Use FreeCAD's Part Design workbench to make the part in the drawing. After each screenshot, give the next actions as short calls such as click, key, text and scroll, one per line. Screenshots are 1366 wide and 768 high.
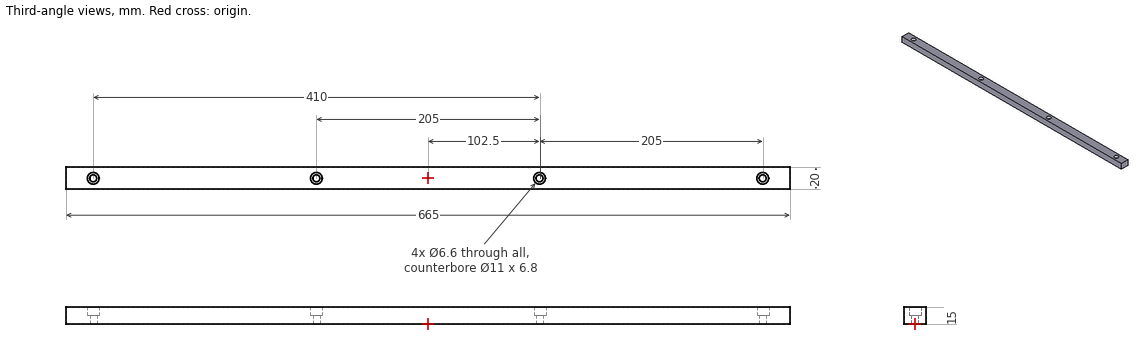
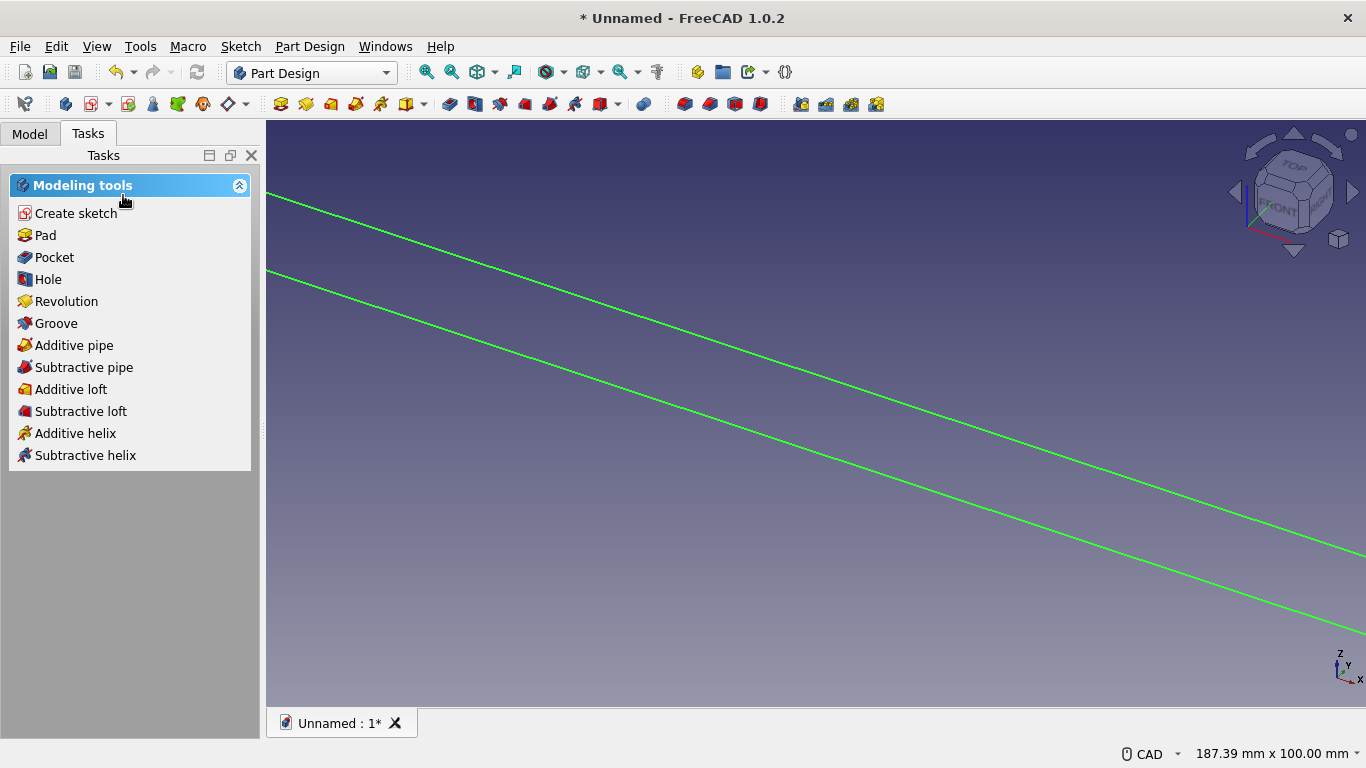
click(281, 104)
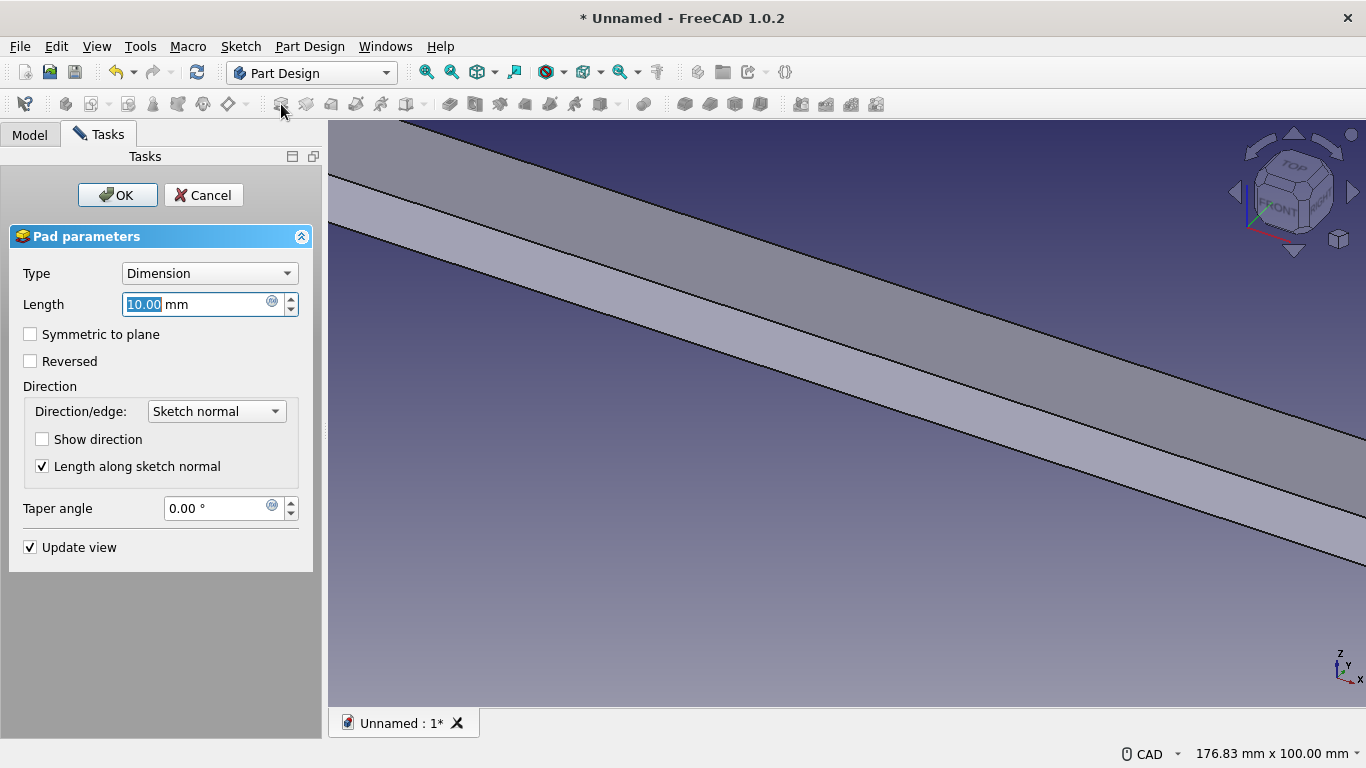
text(15)
key(Tab)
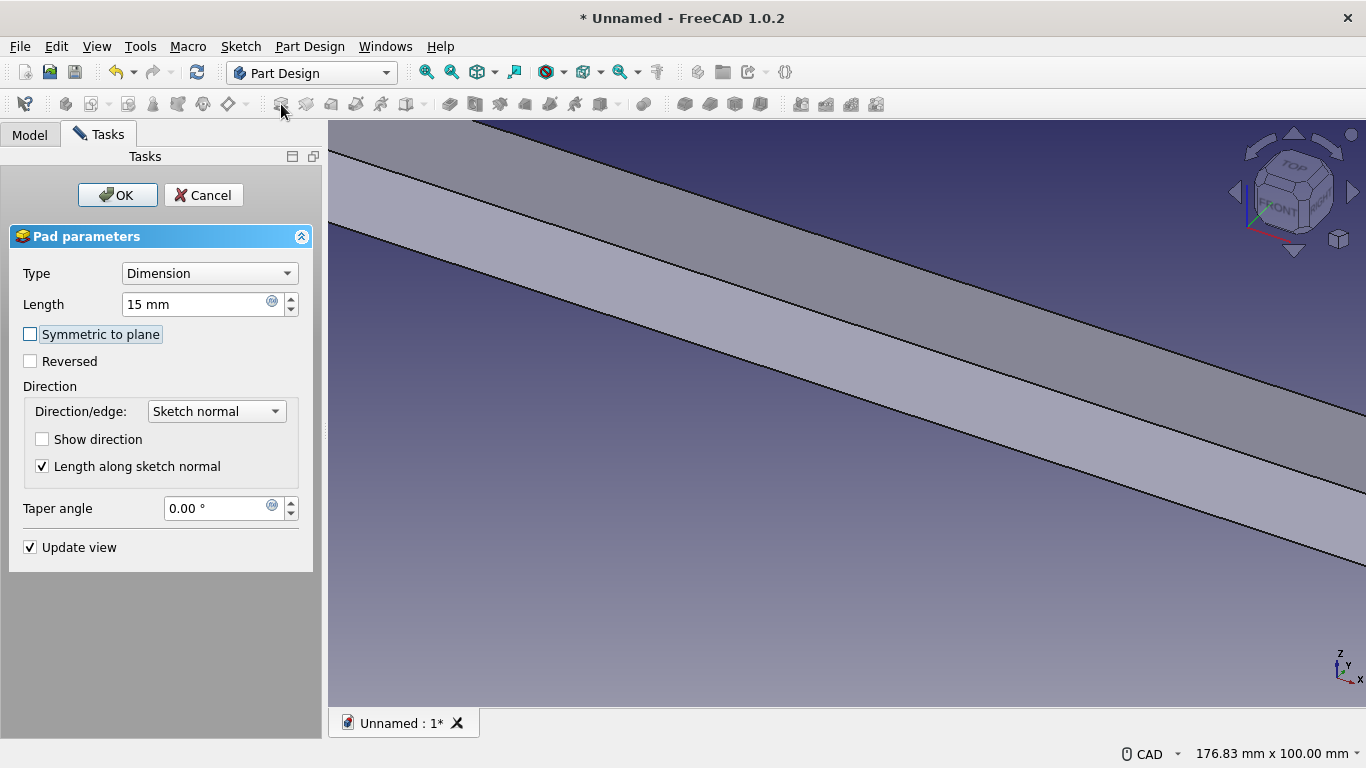
click(118, 195)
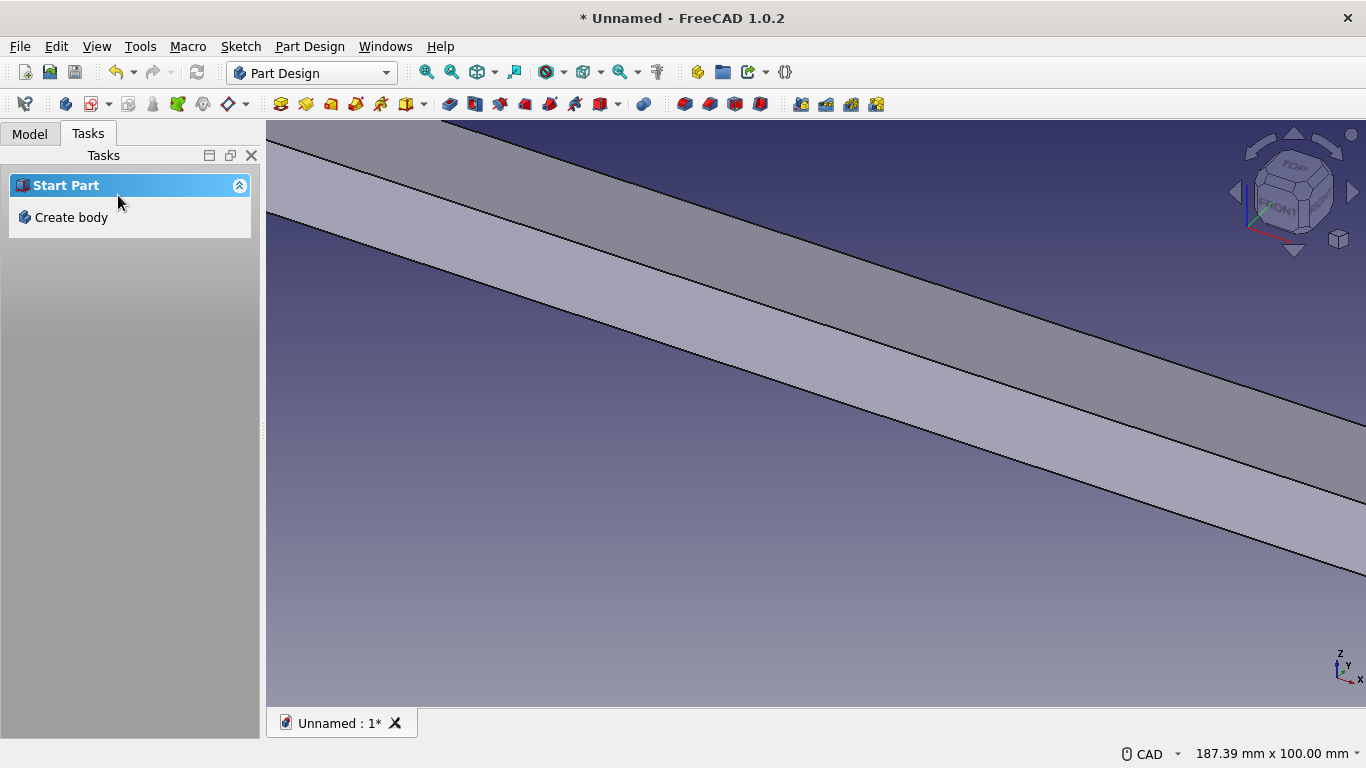
click(427, 72)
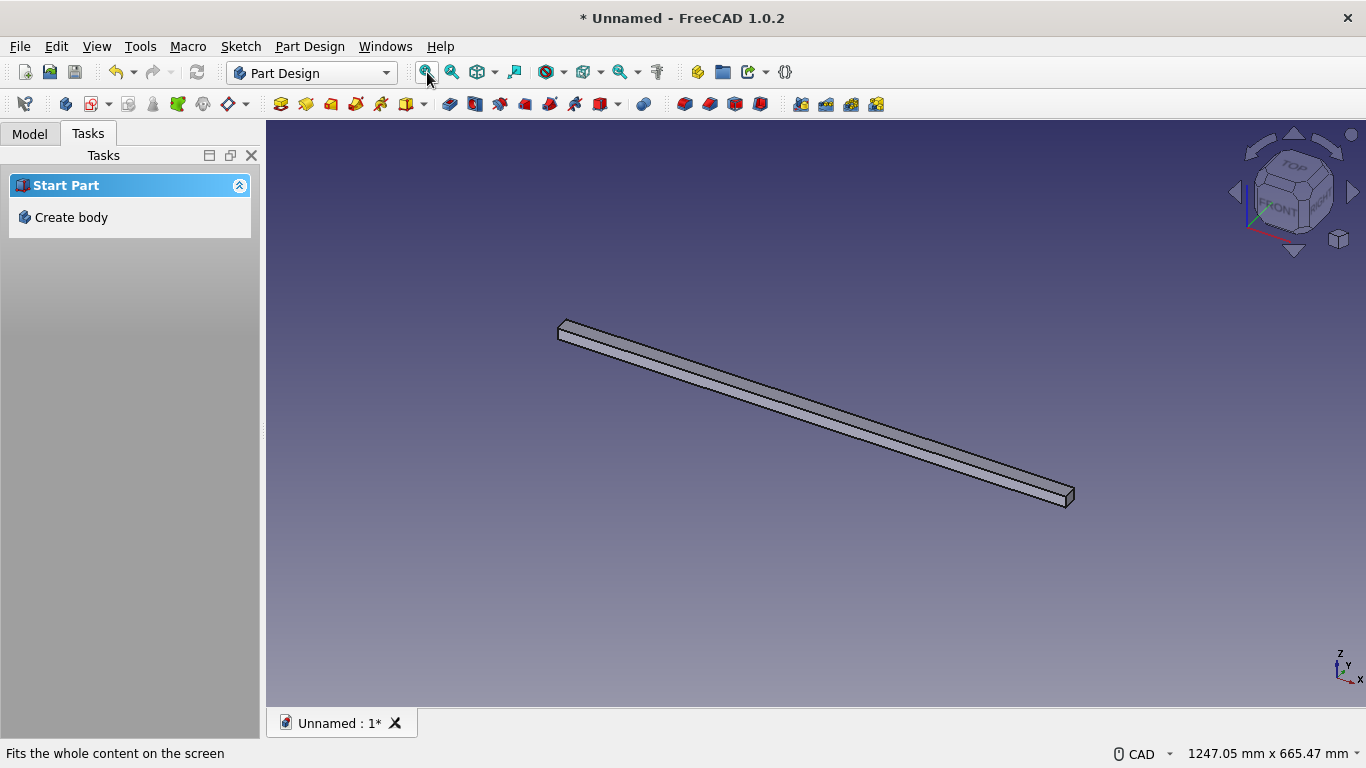
key(0)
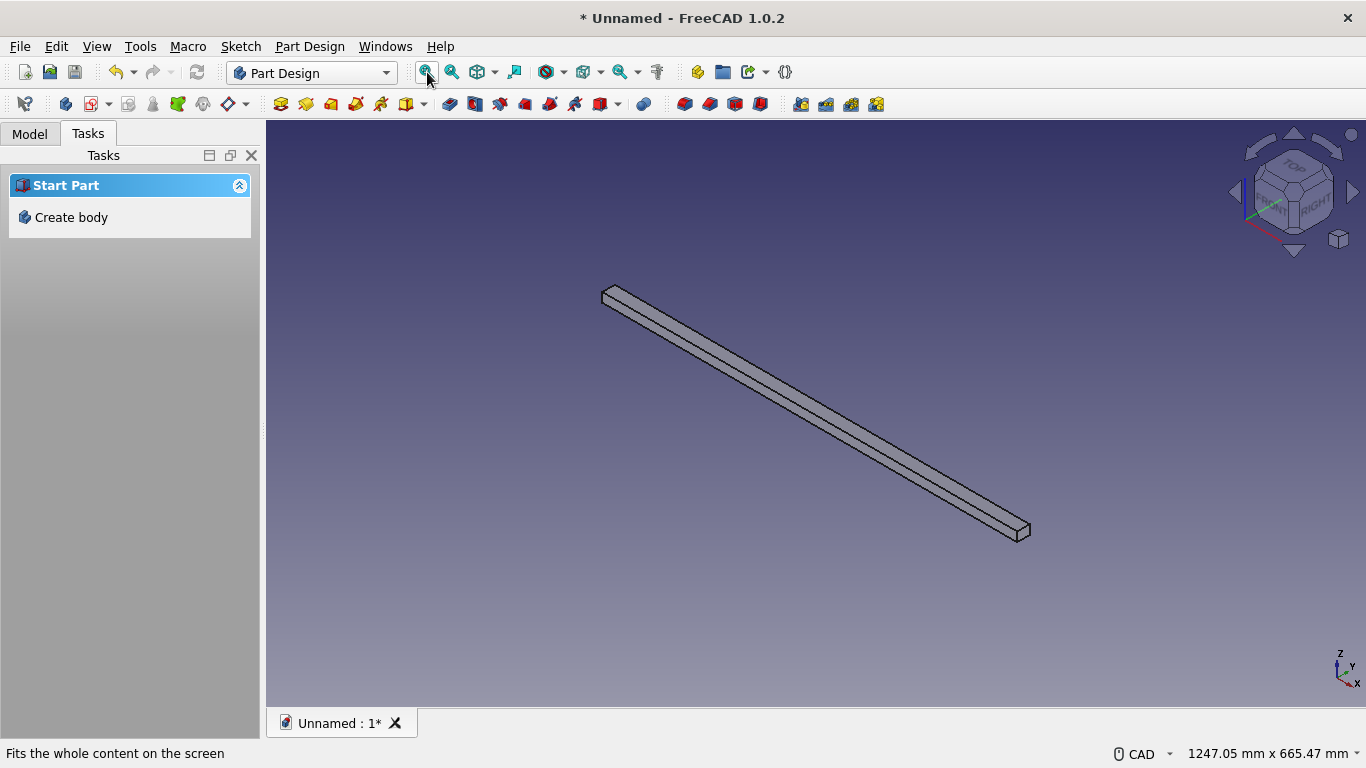
click(427, 72)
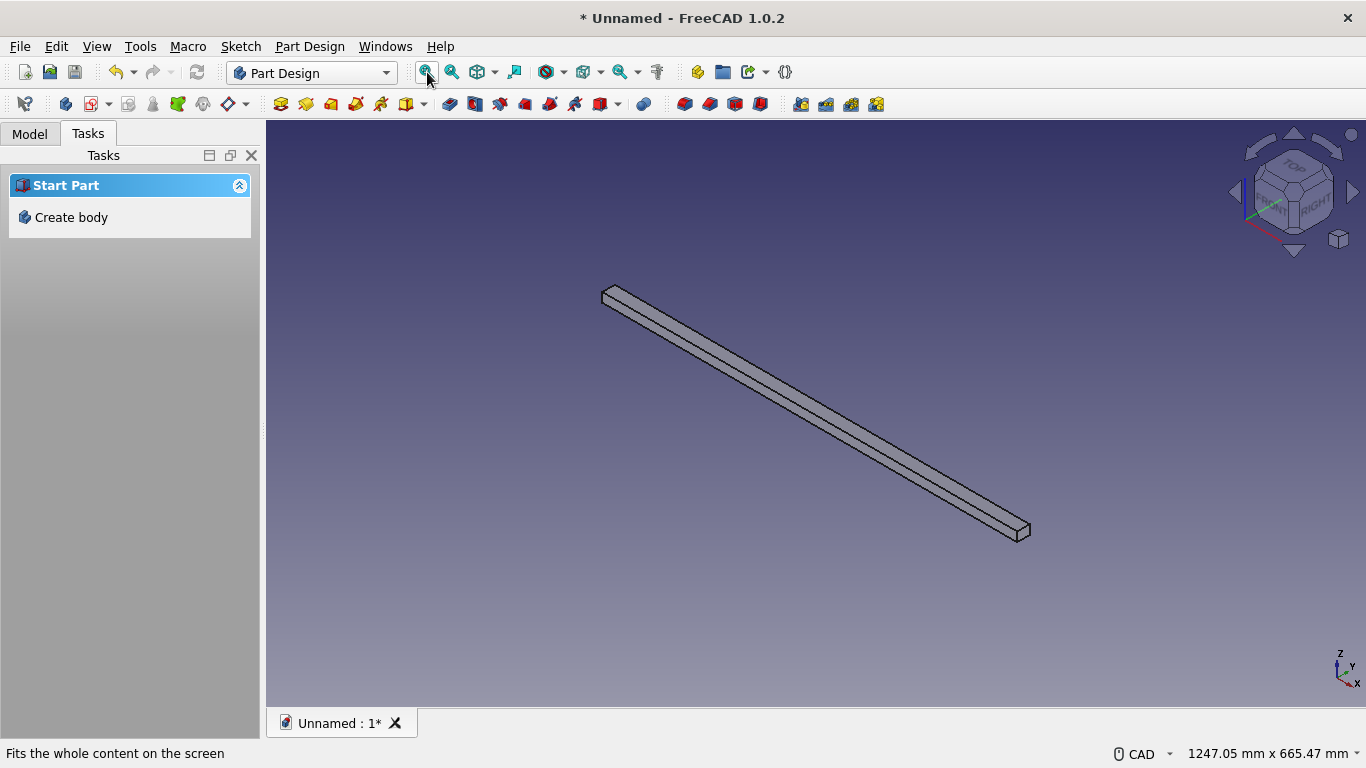
key(2)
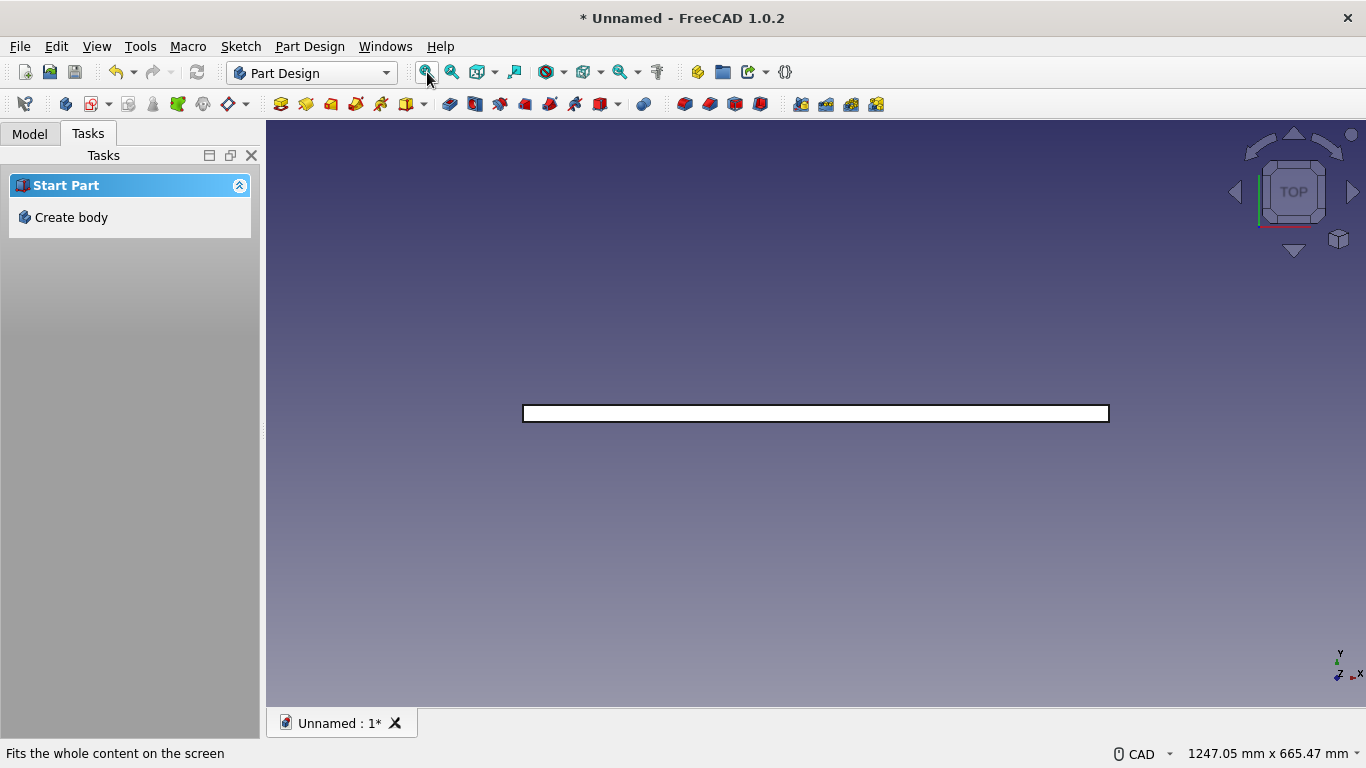
click(1067, 412)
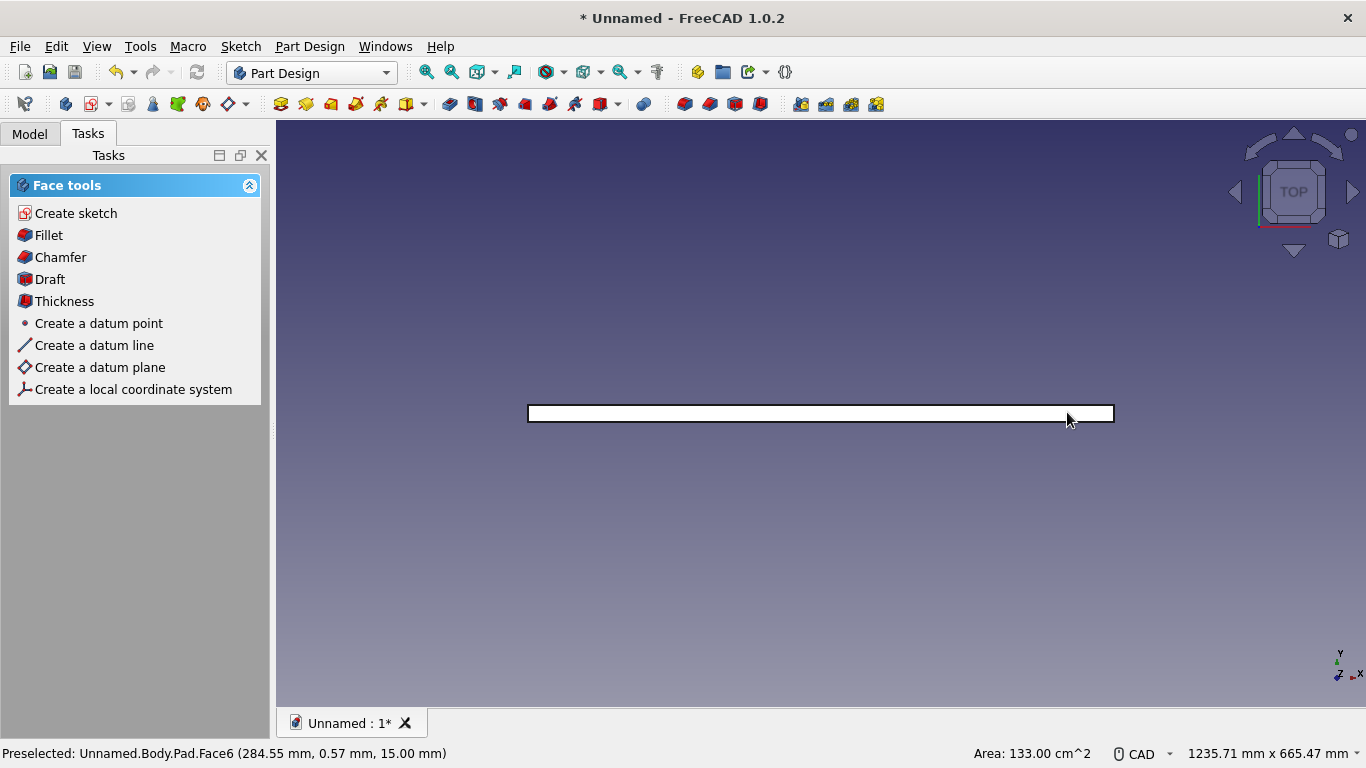
click(90, 104)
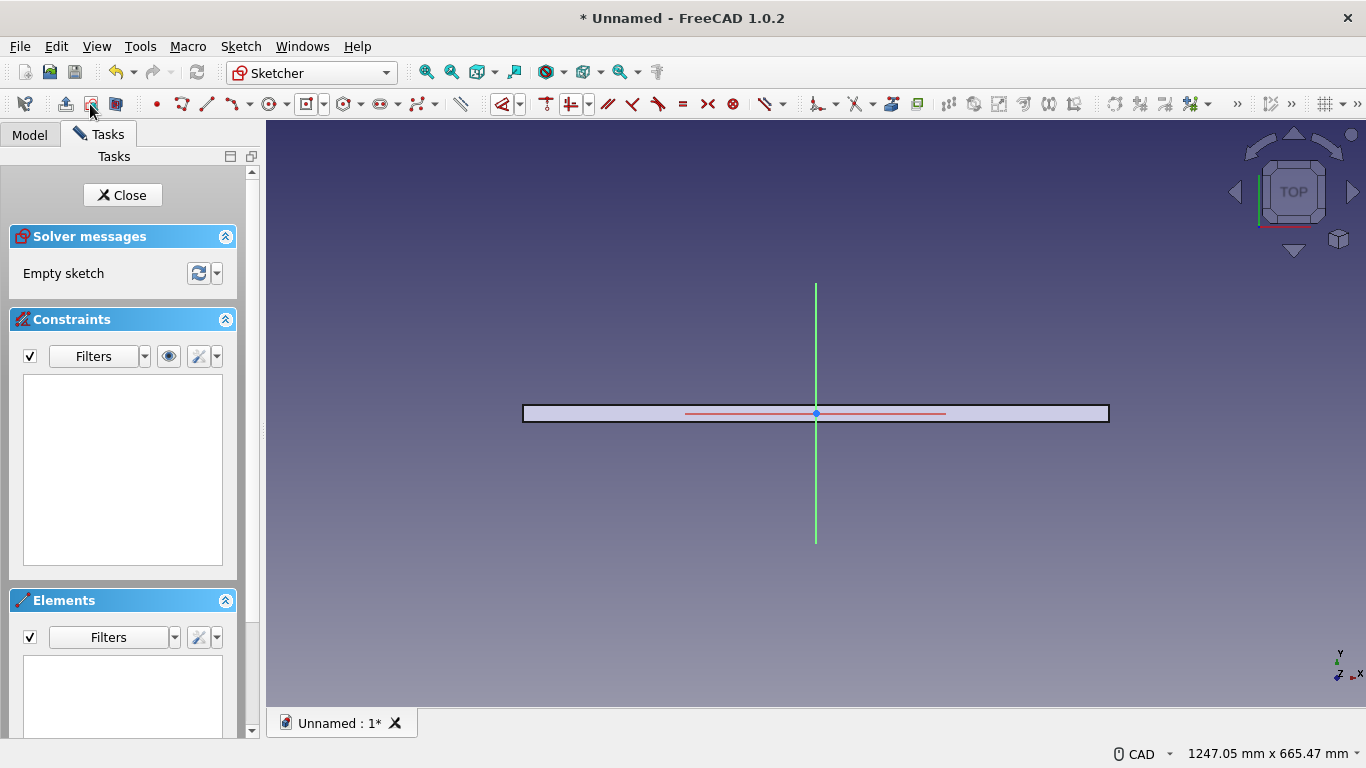
click(268, 104)